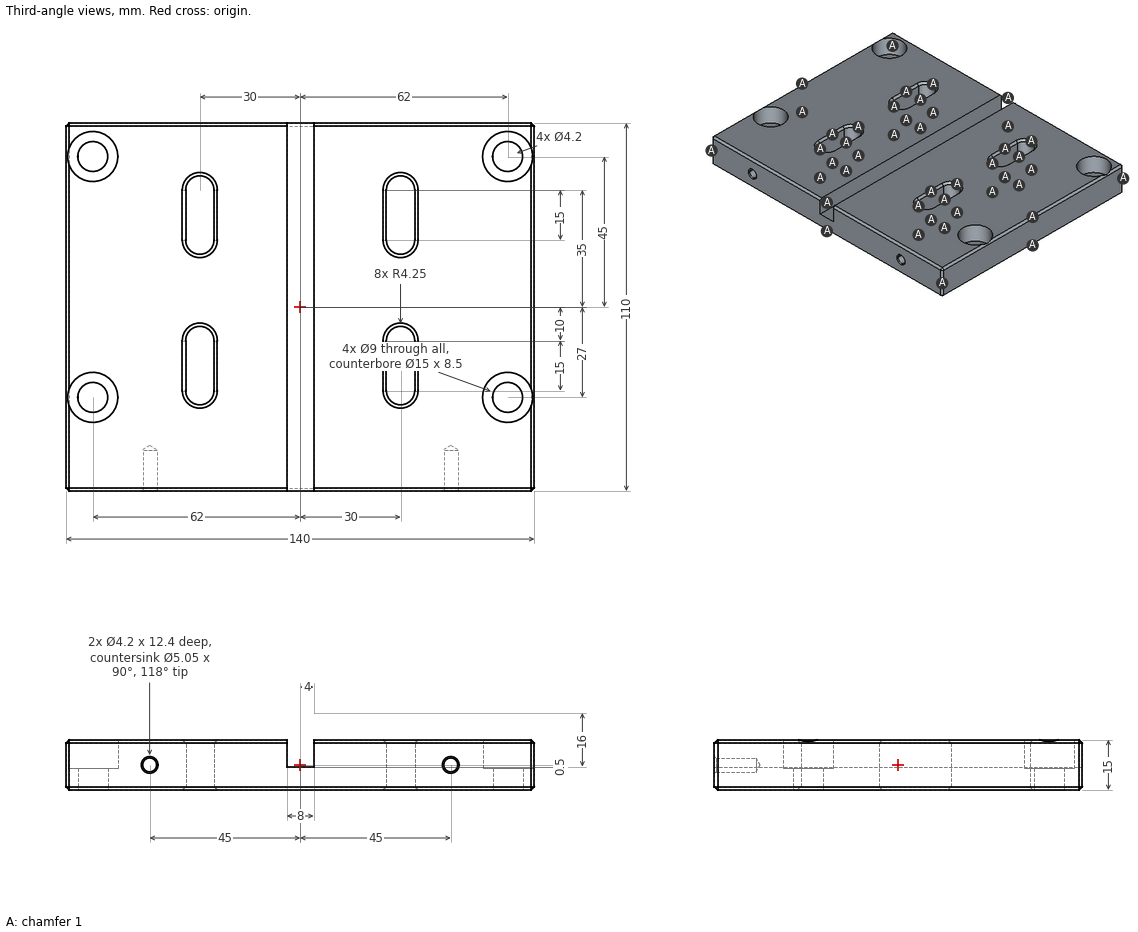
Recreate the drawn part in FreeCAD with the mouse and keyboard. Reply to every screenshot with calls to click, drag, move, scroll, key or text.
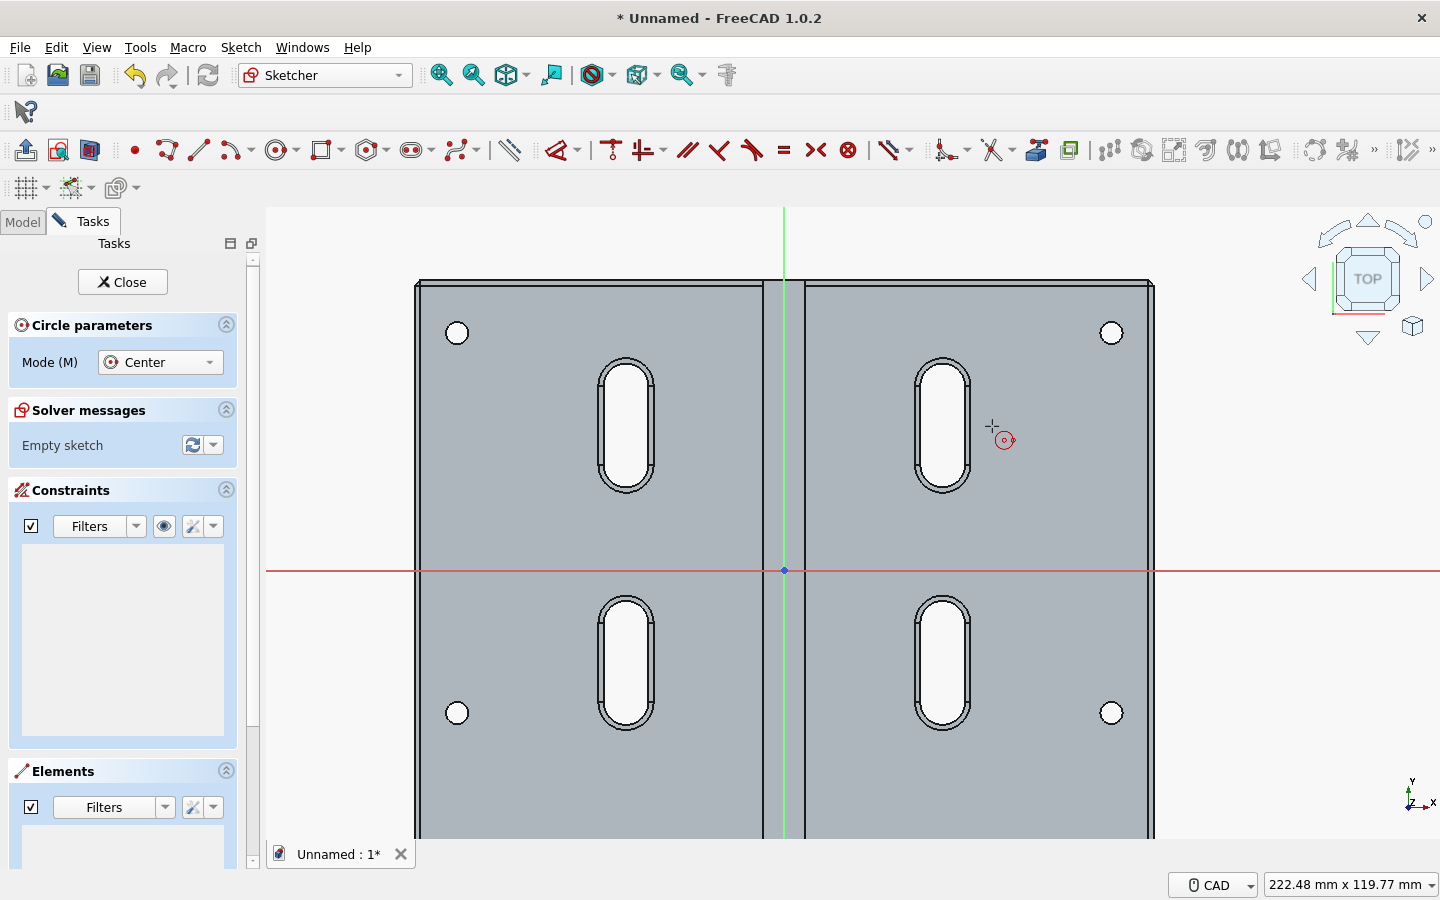
click(1111, 713)
click(1128, 696)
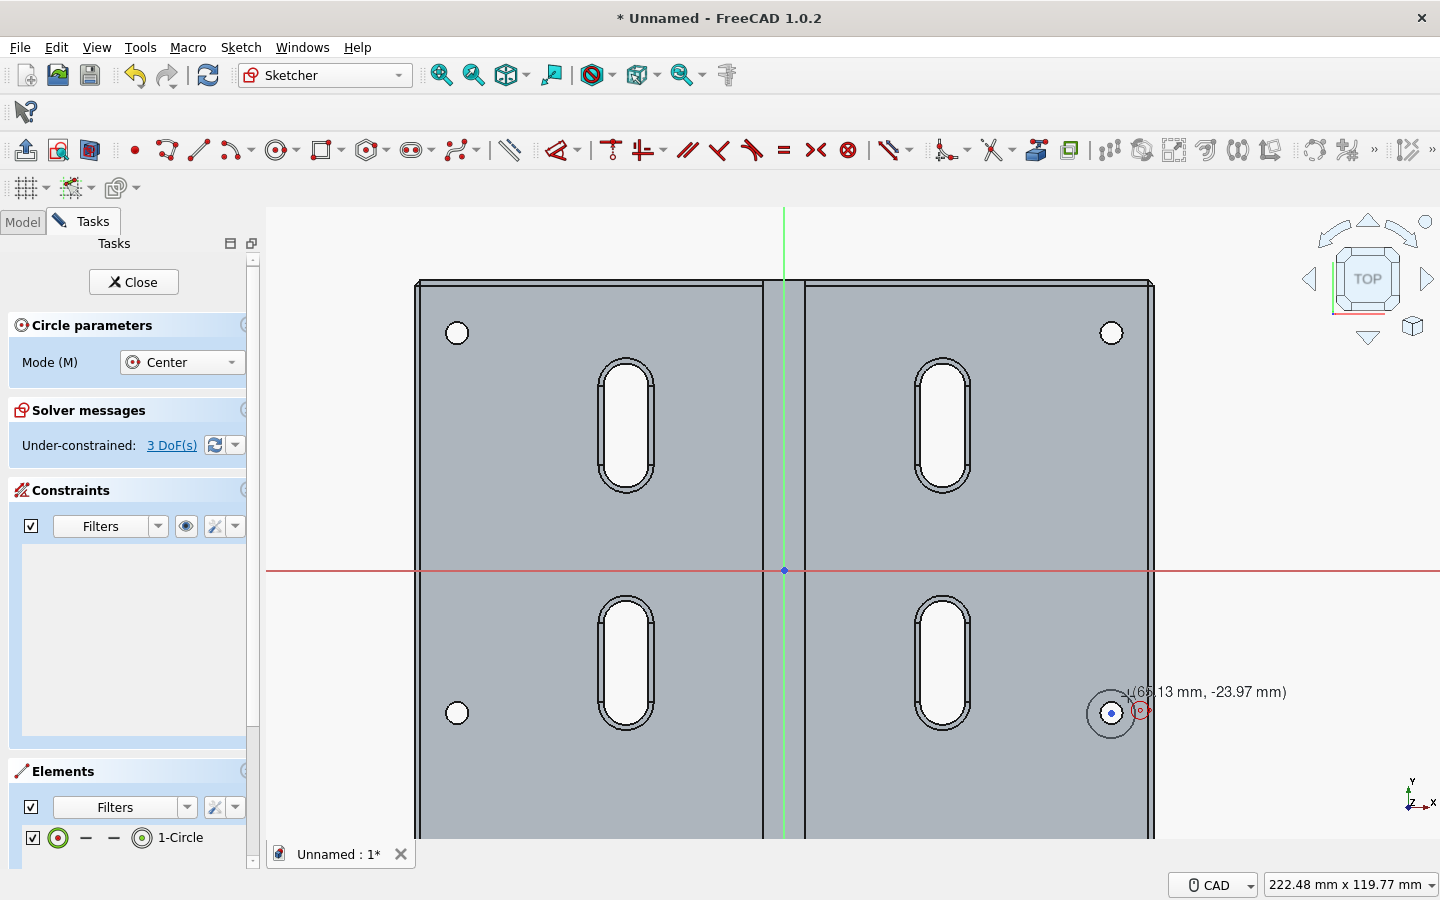
click(1111, 333)
click(1128, 316)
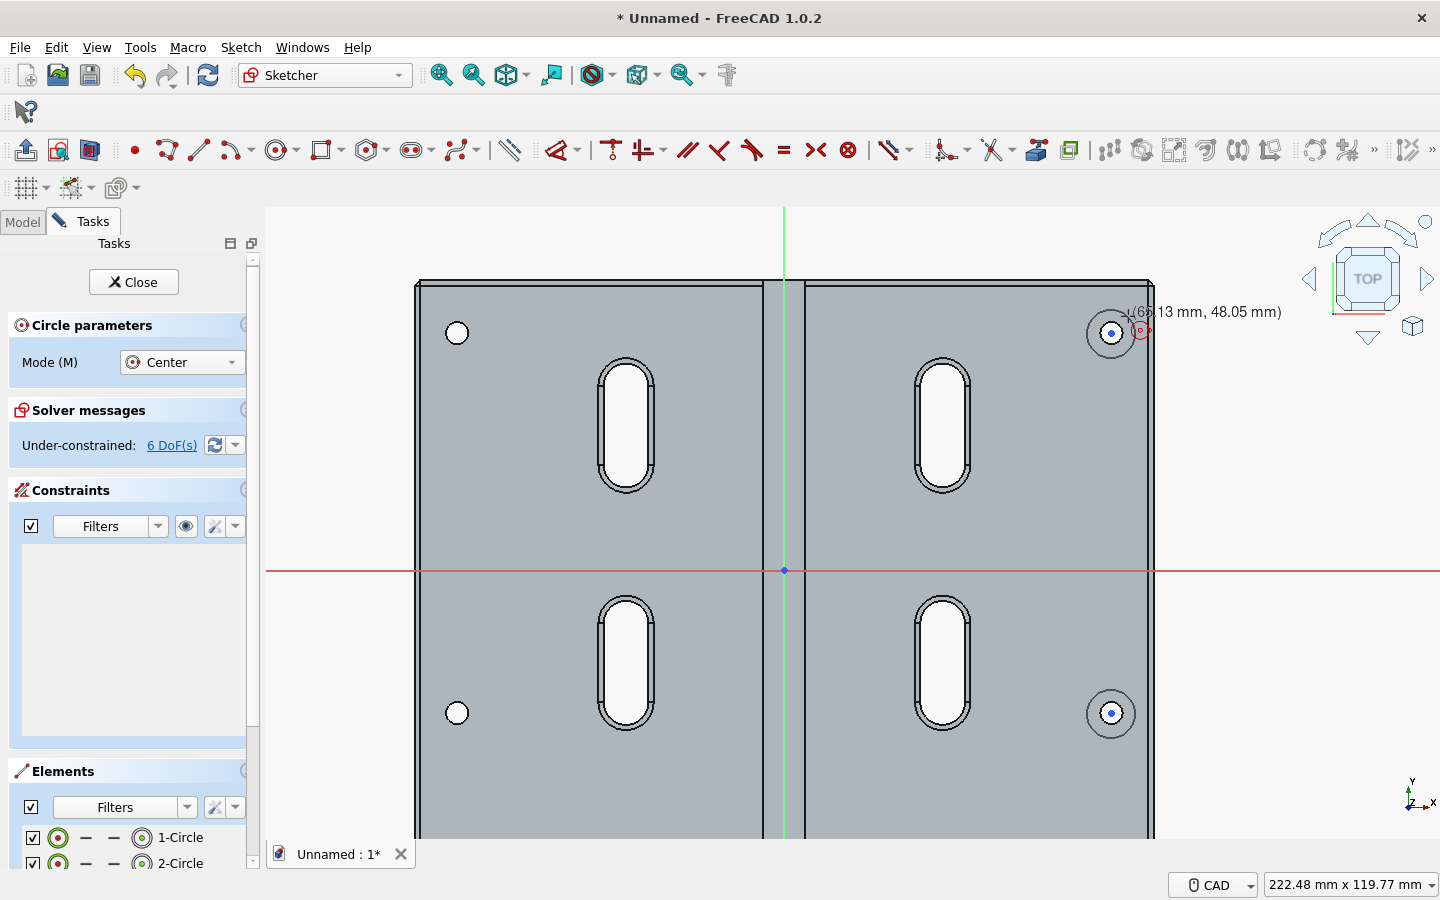
click(457, 333)
click(474, 316)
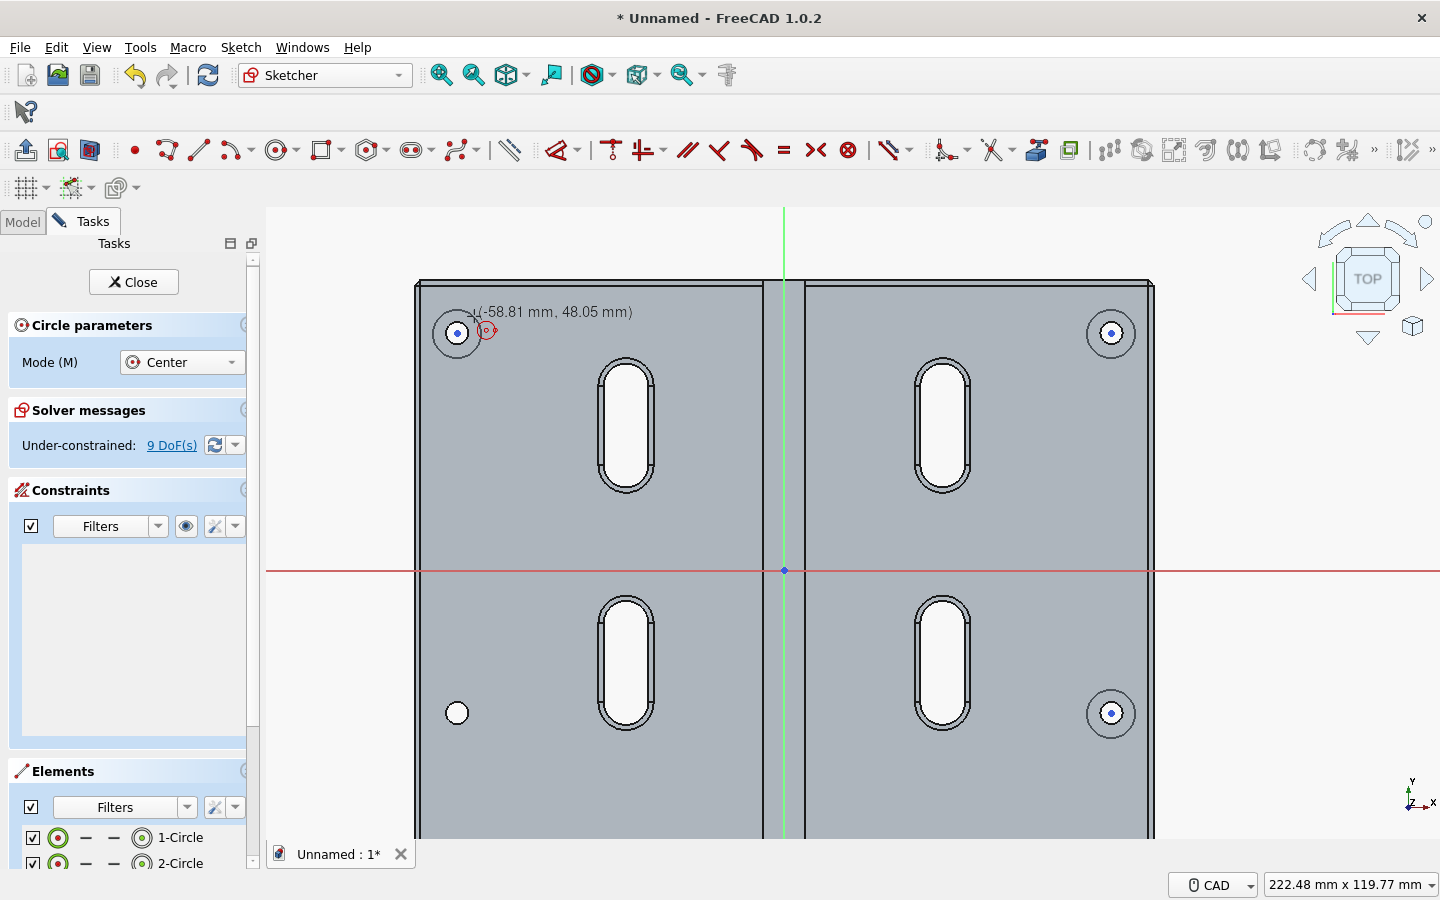
click(457, 713)
click(474, 696)
key(Escape)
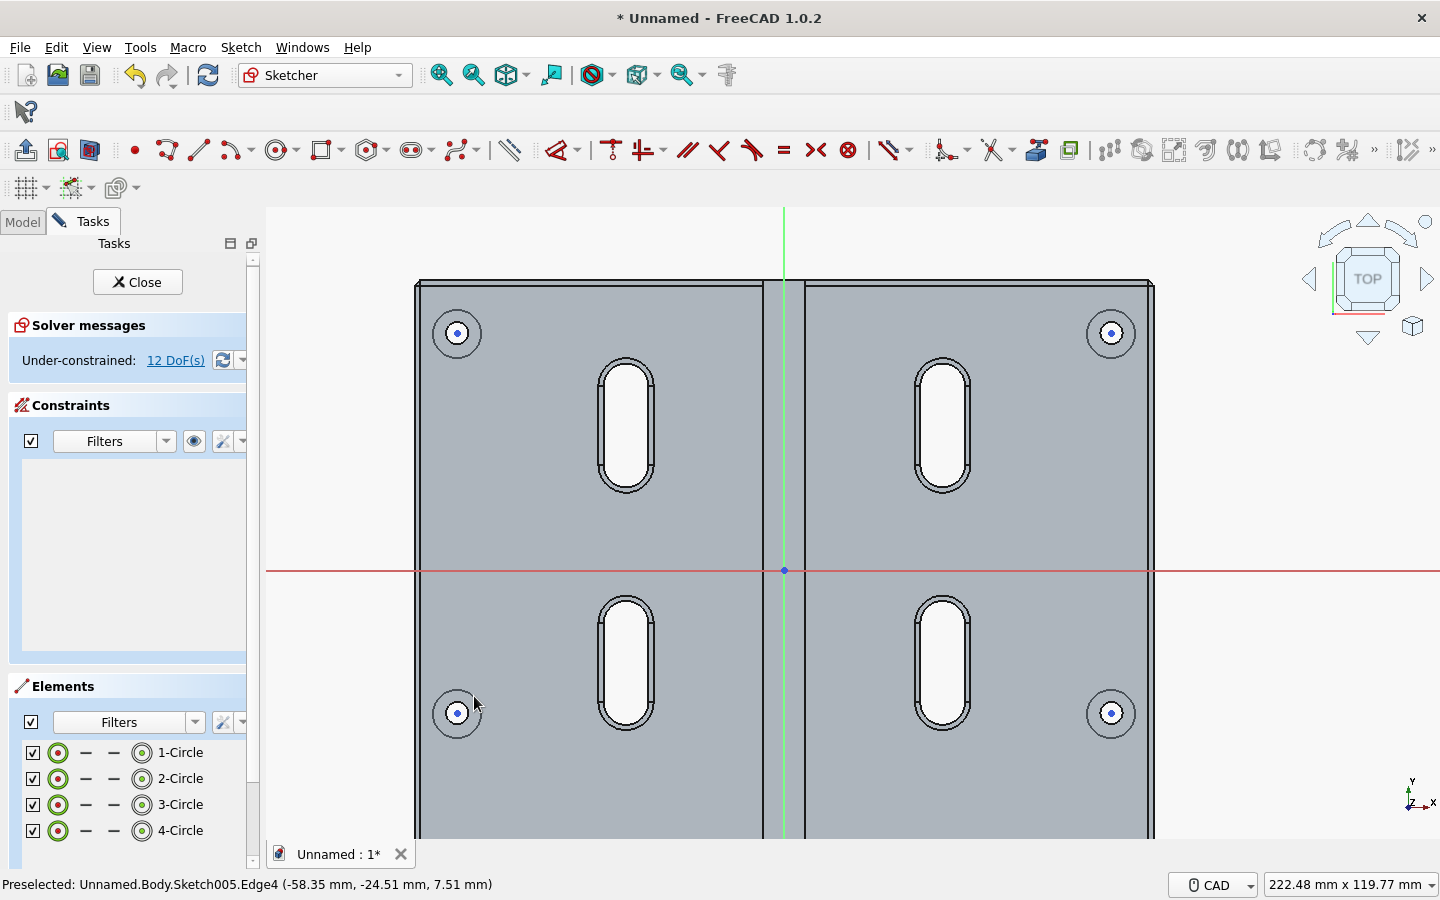
click(1128, 697)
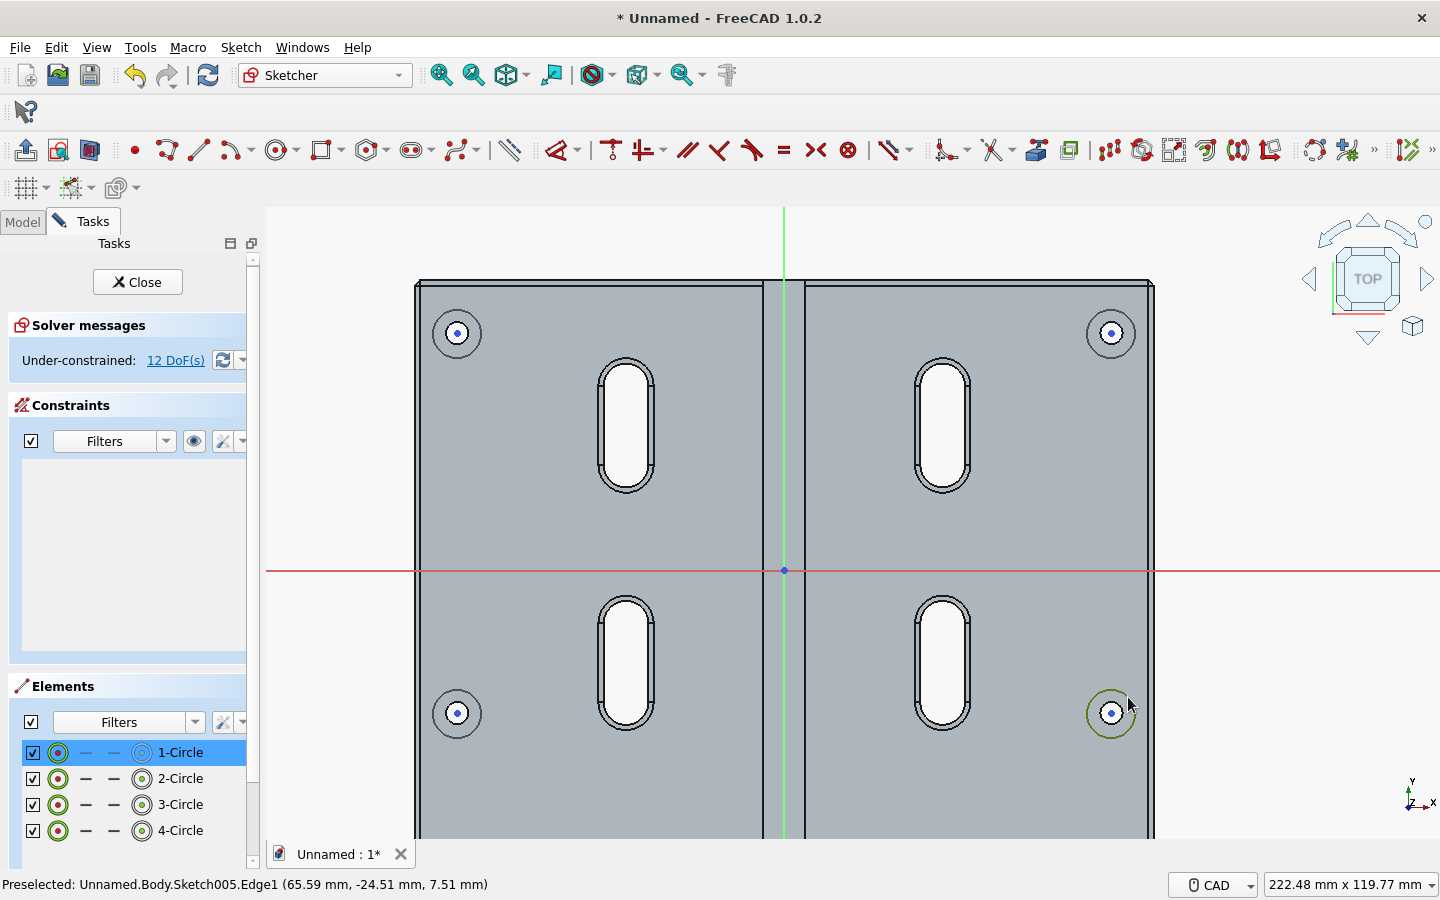
click(1128, 317)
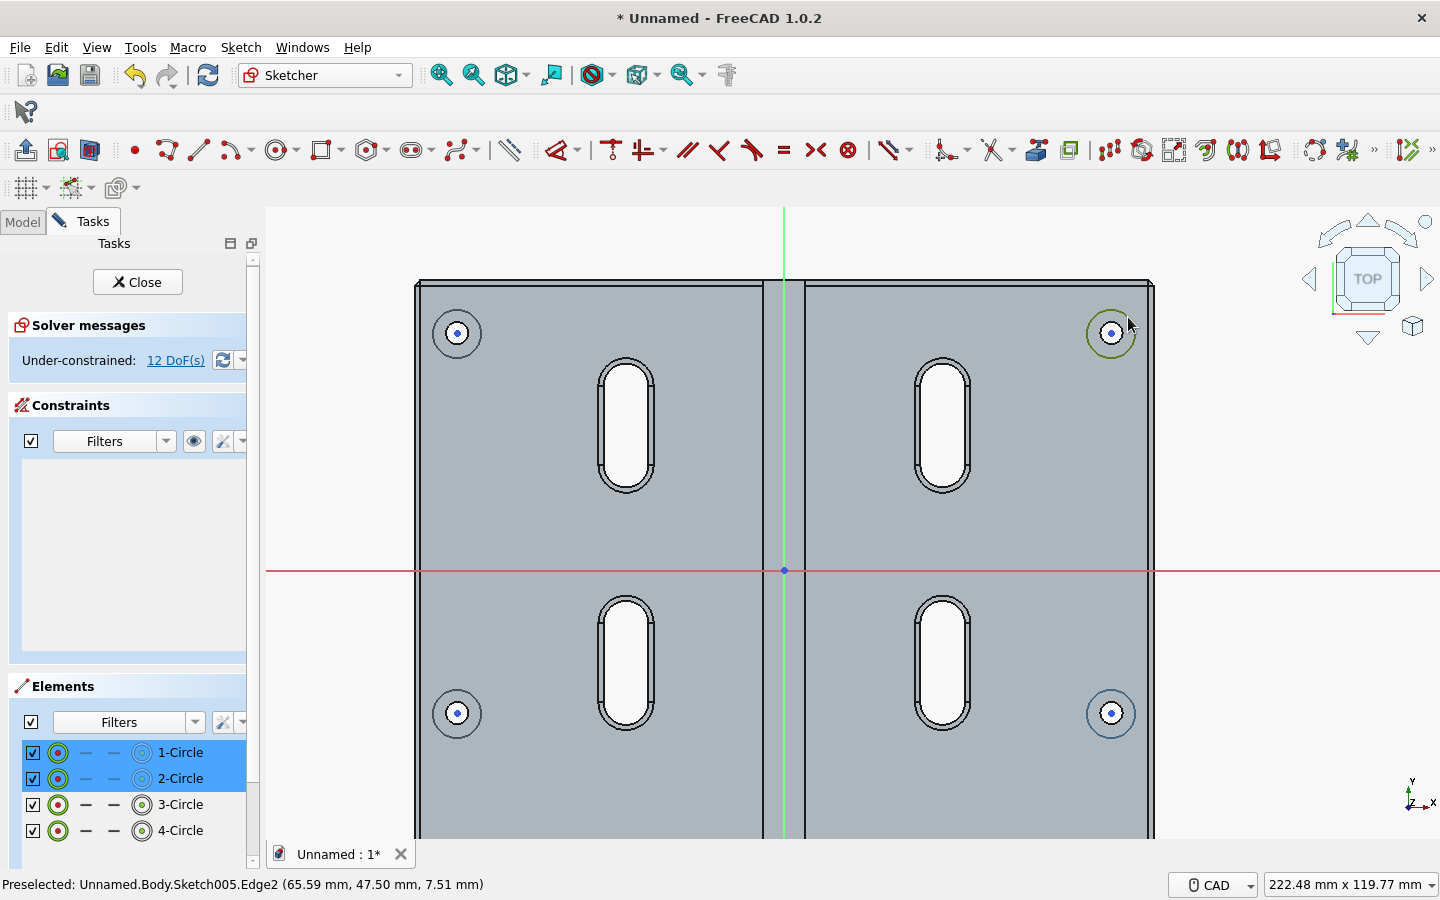
click(474, 317)